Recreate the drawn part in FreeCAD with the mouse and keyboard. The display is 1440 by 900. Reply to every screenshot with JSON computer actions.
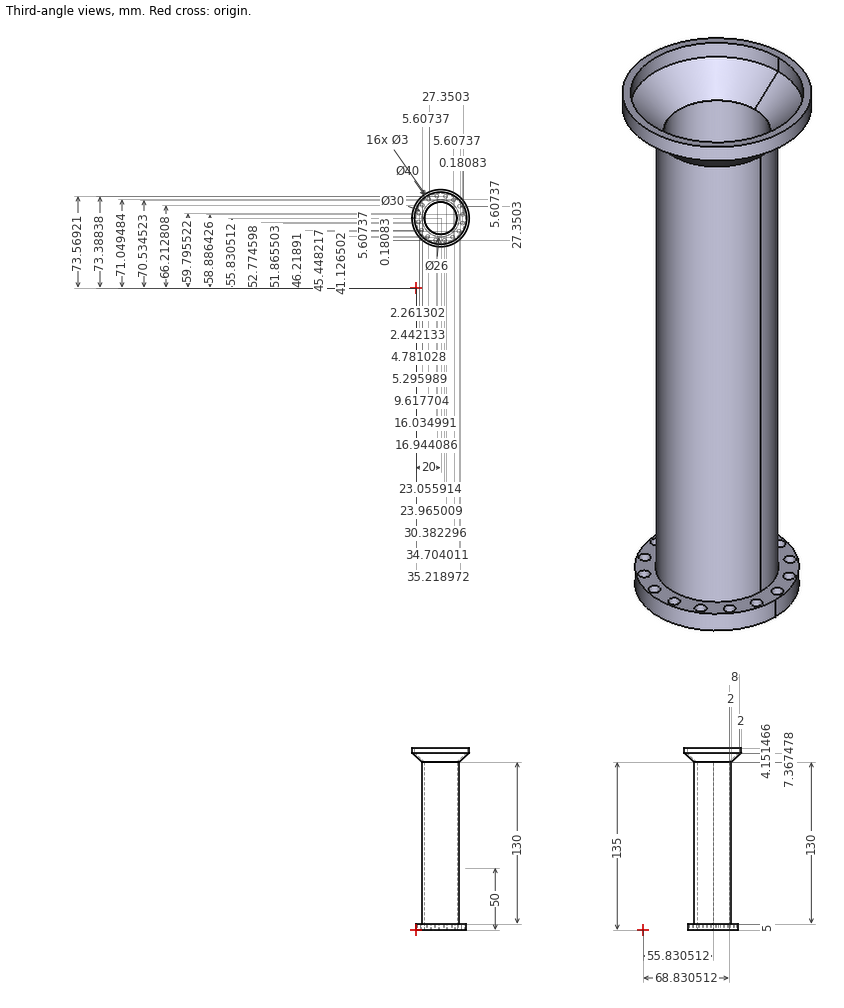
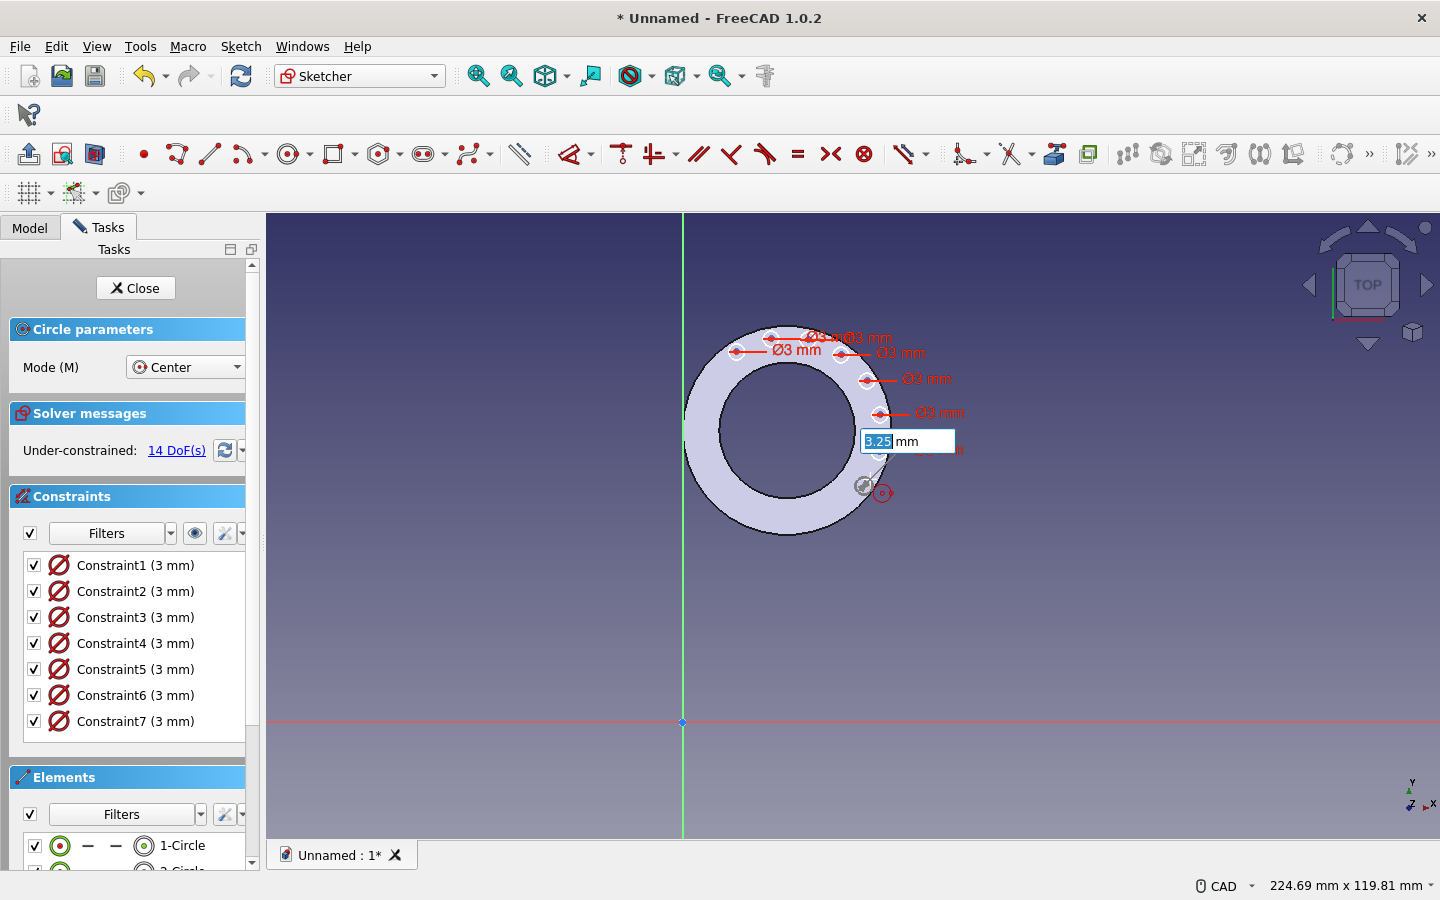
{"action": "type", "text": "3"}
{"action": "key", "text": "Return"}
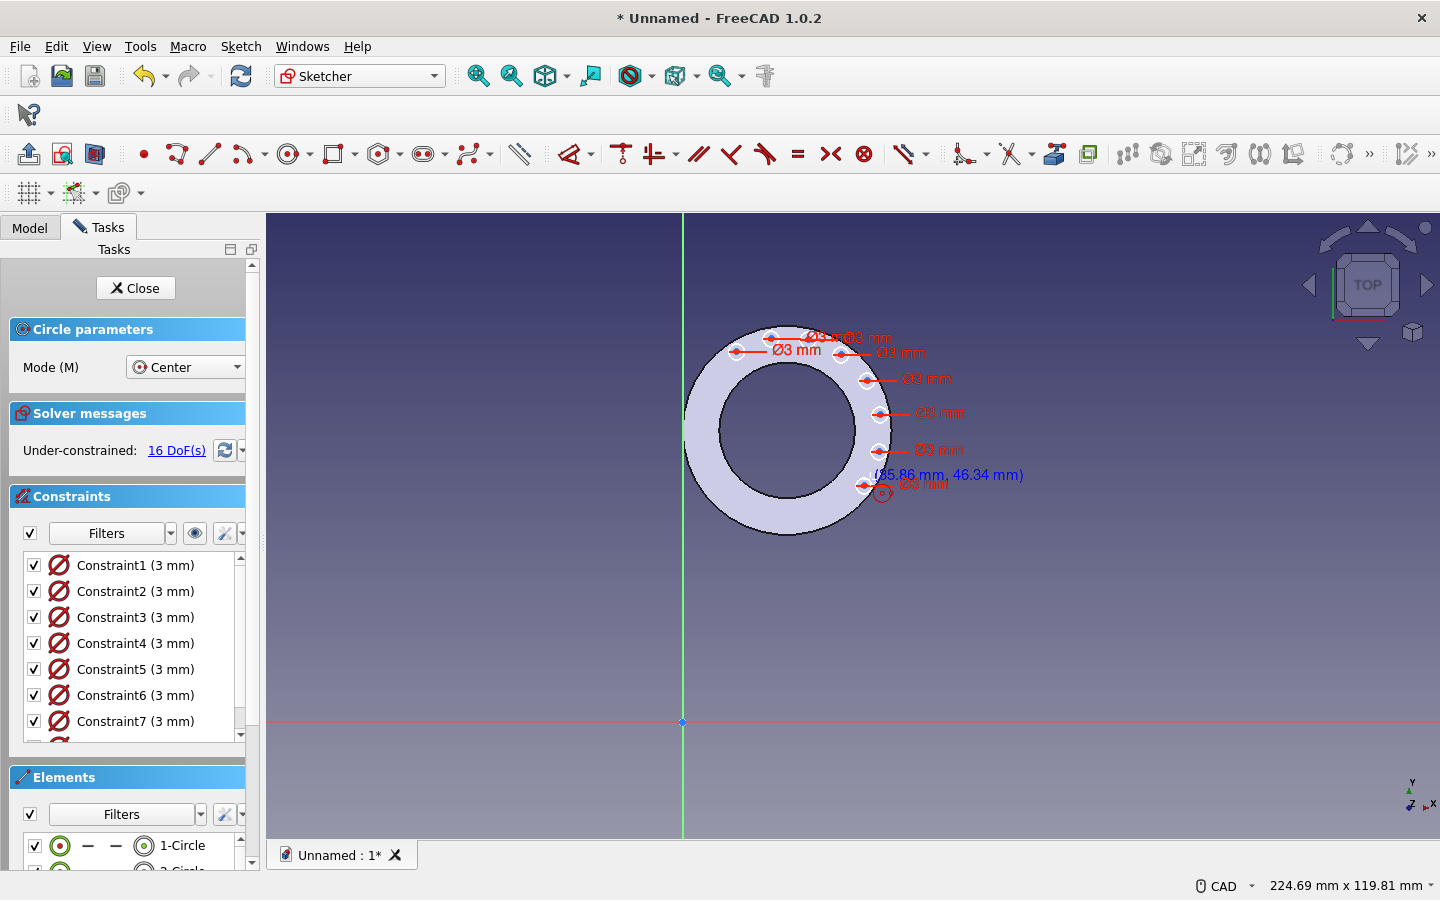
{"action": "scroll", "coordinate": [837, 510], "scroll_direction": "up", "scroll_amount": 6}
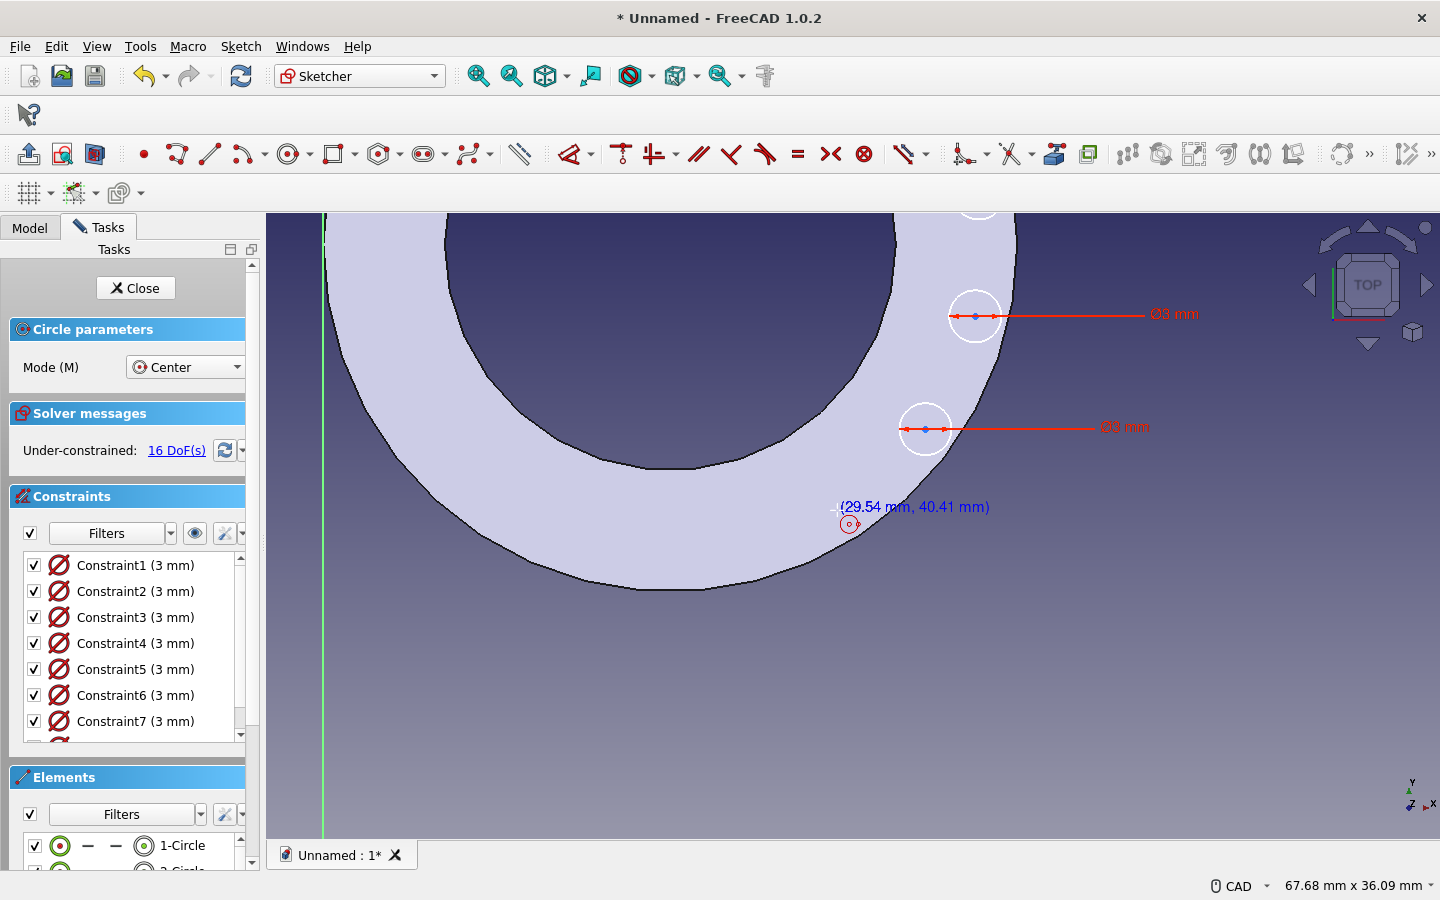
{"action": "scroll", "coordinate": [837, 510], "scroll_direction": "down", "scroll_amount": 6}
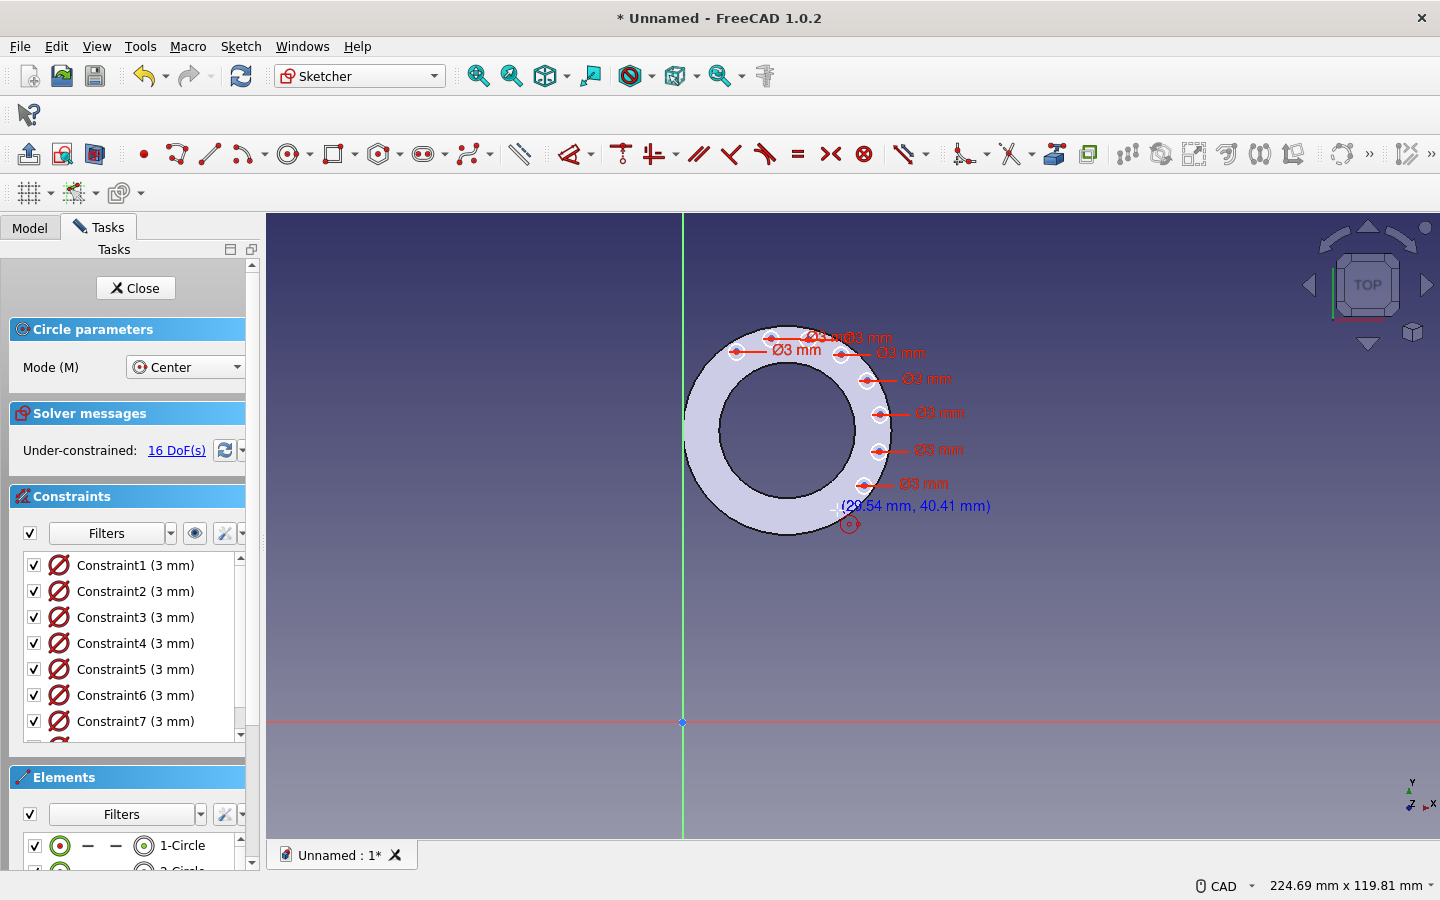
{"action": "left_click", "coordinate": [837, 510]}
{"action": "mouse_move", "coordinate": [843, 504]}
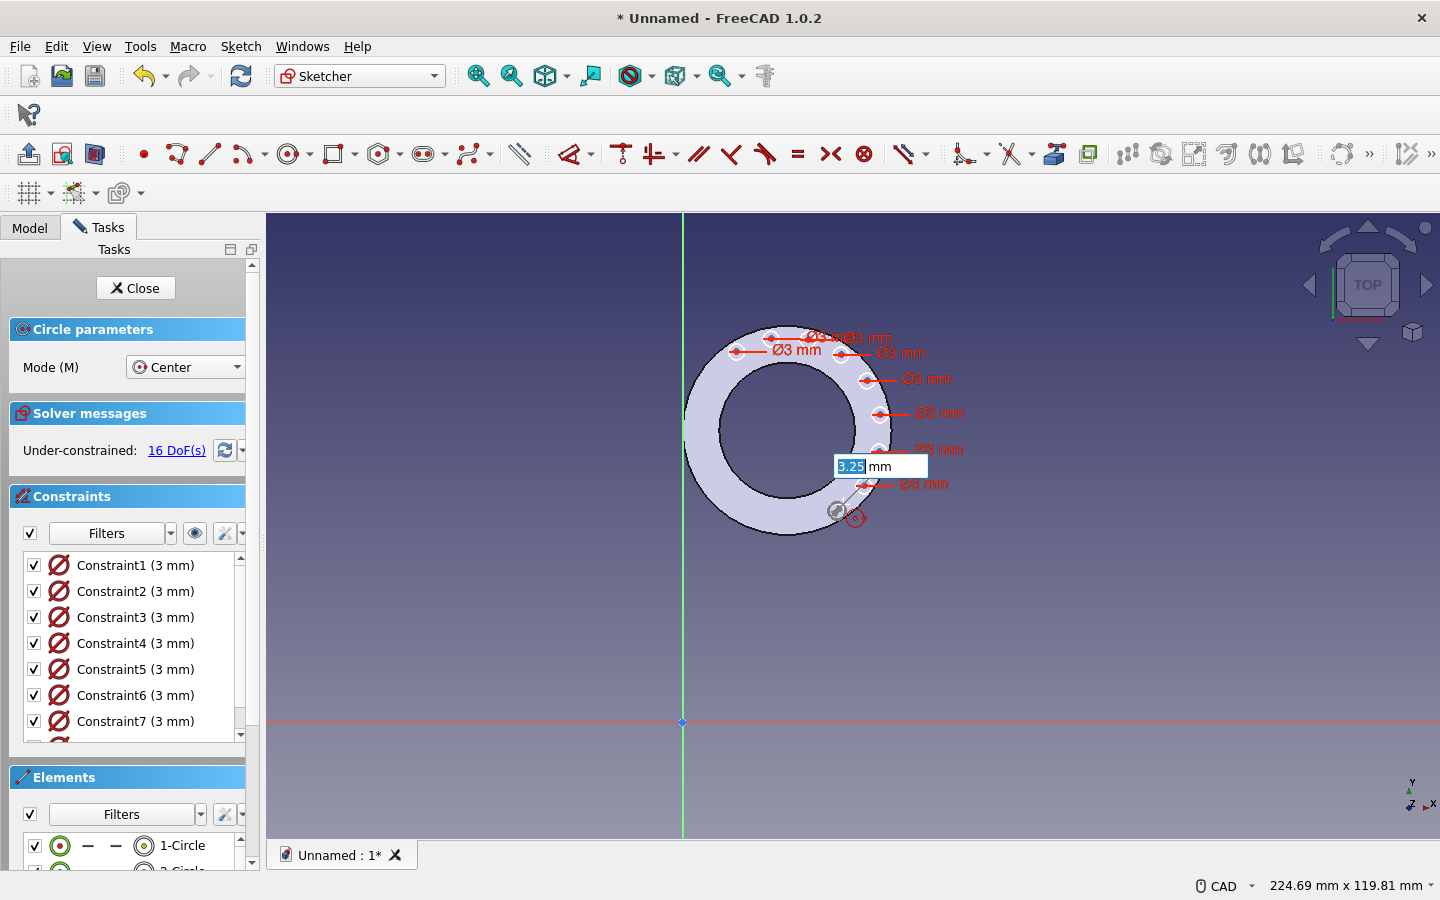
{"action": "type", "text": "3"}
{"action": "key", "text": "Return"}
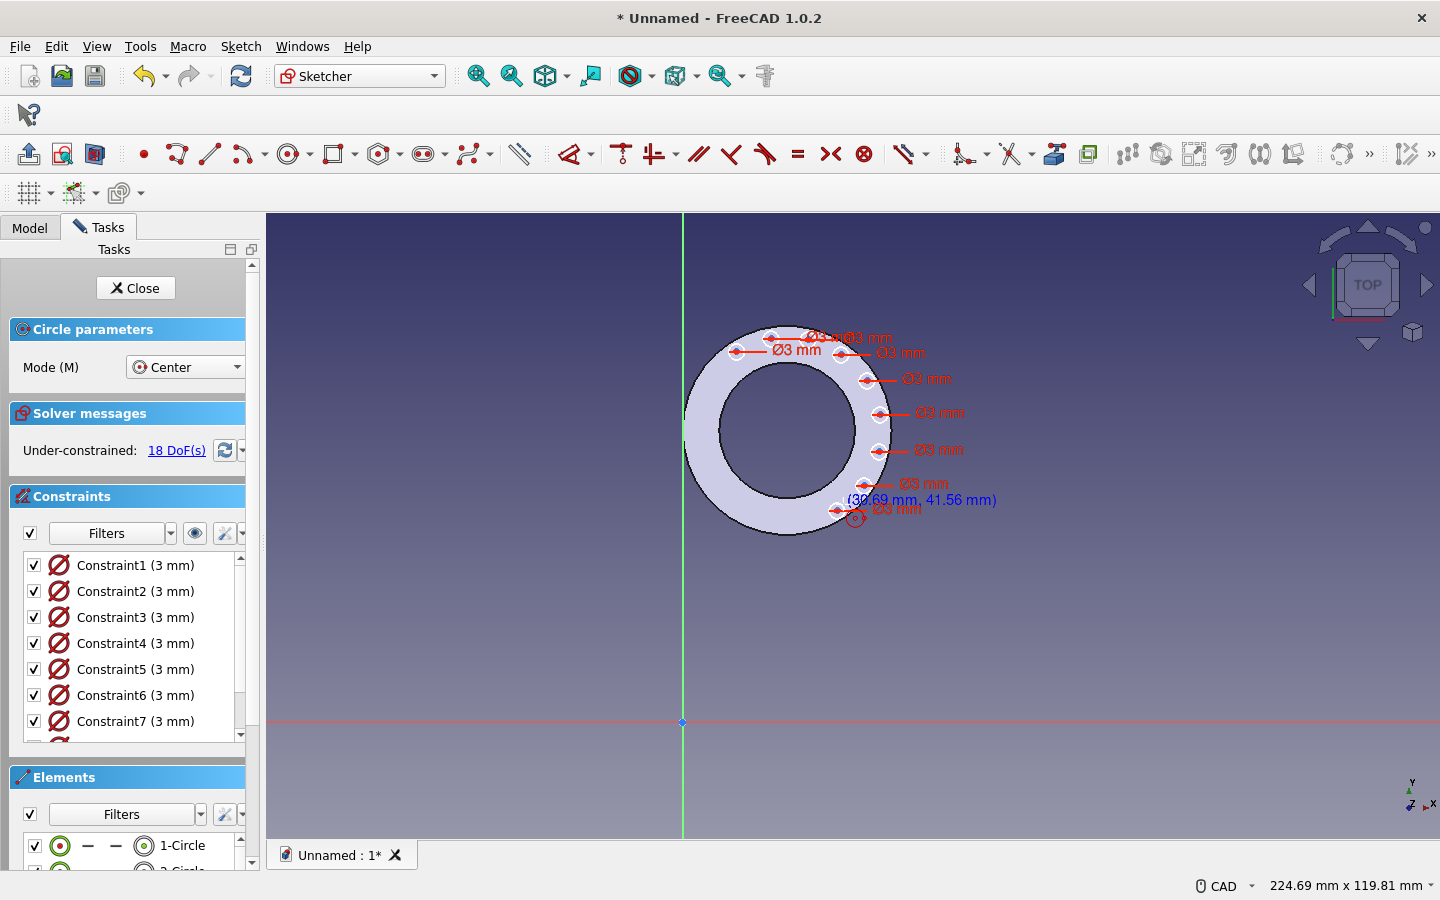
{"action": "scroll", "coordinate": [803, 523], "scroll_direction": "up", "scroll_amount": 6}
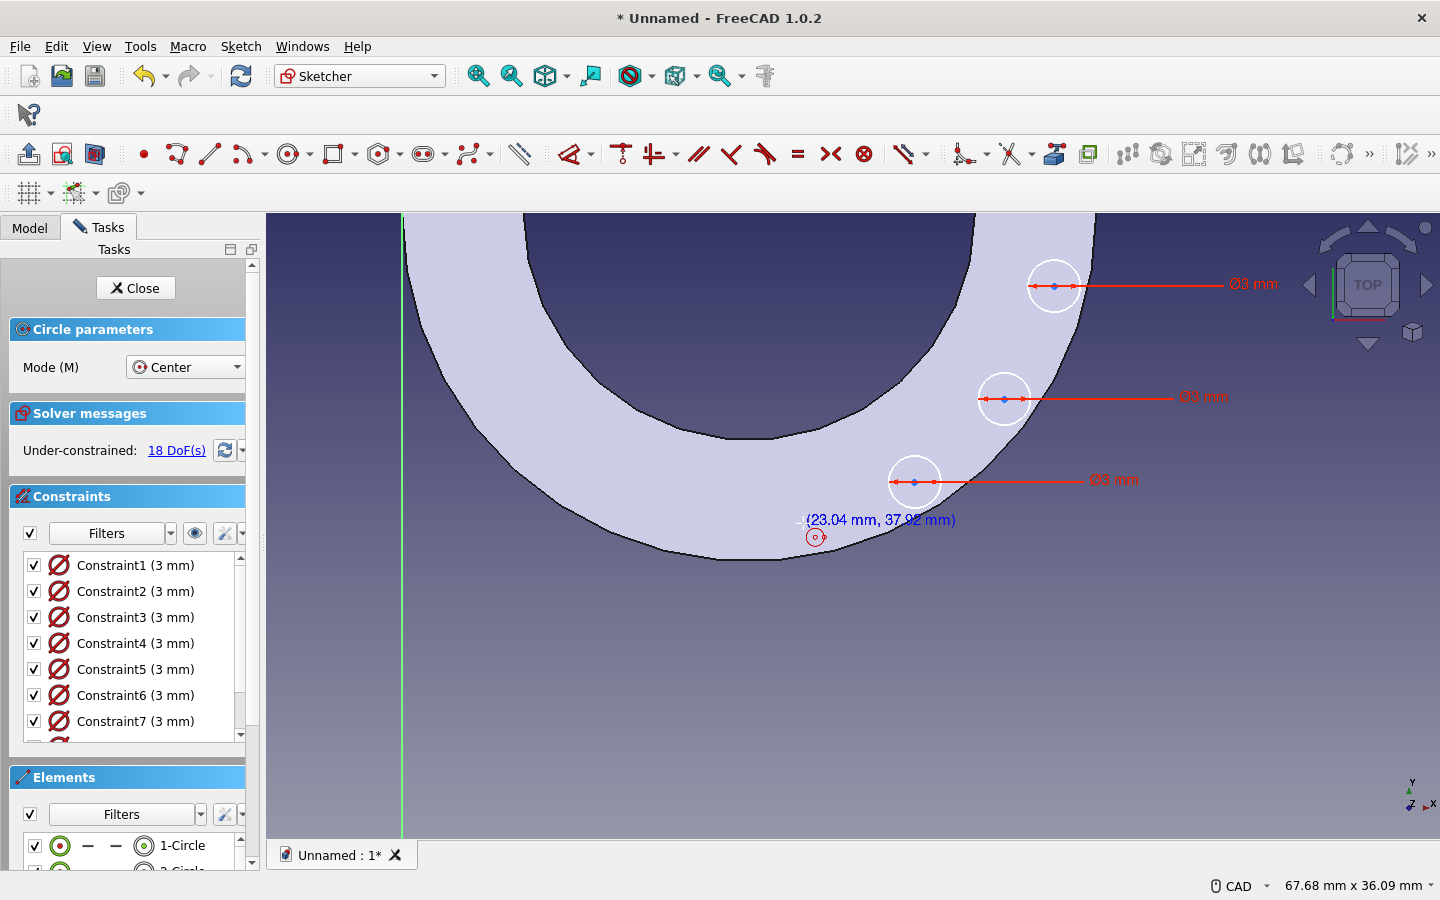
{"action": "scroll", "coordinate": [803, 523], "scroll_direction": "down", "scroll_amount": 6}